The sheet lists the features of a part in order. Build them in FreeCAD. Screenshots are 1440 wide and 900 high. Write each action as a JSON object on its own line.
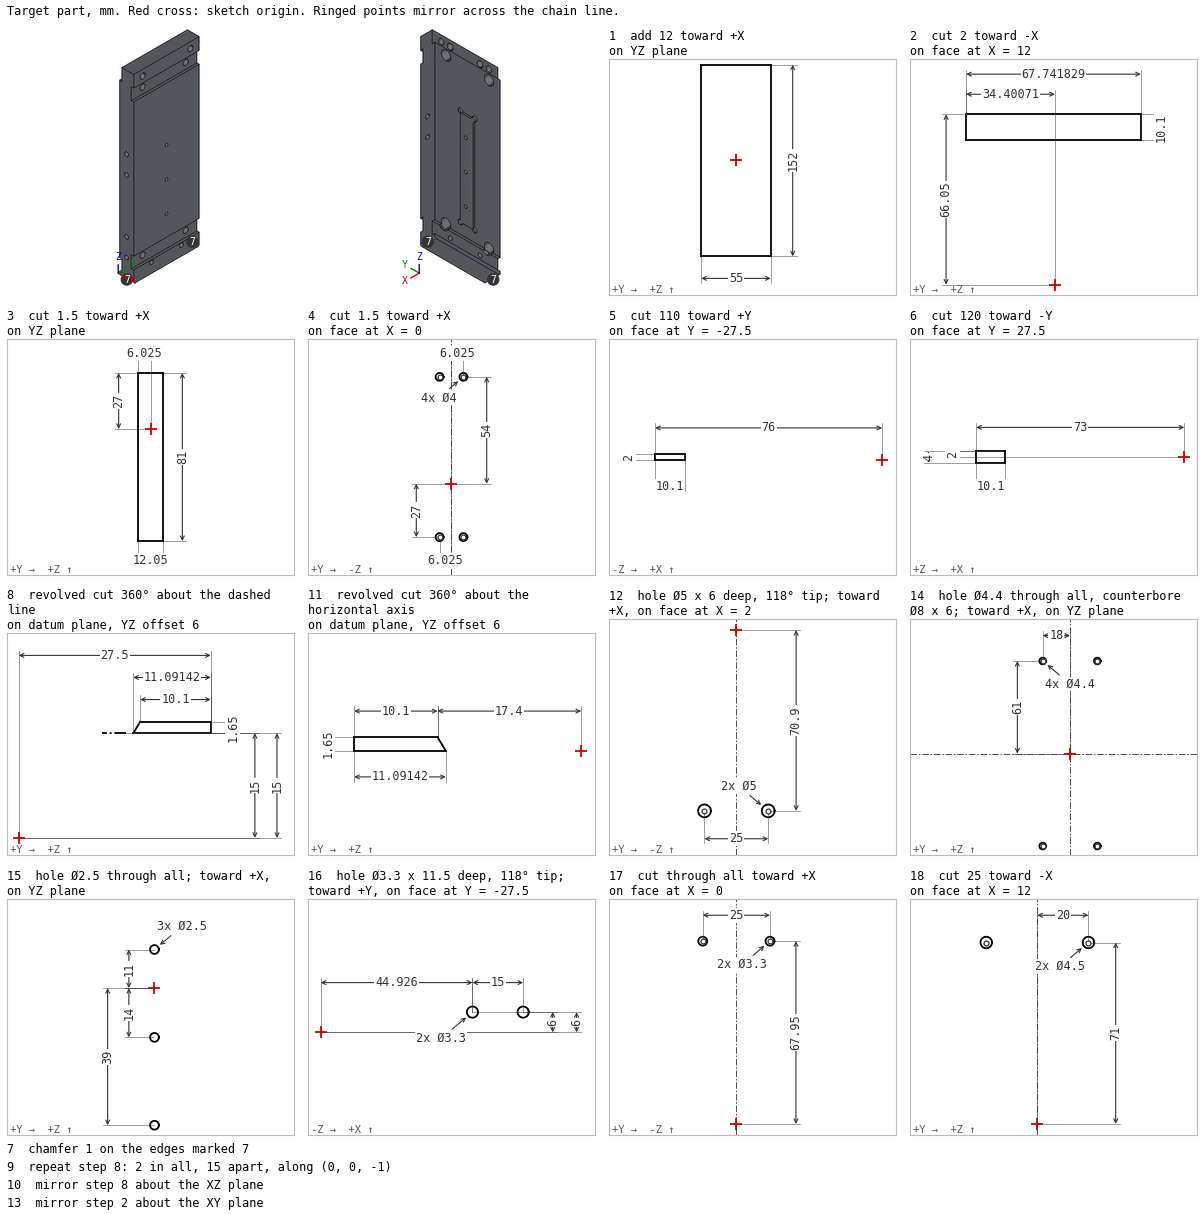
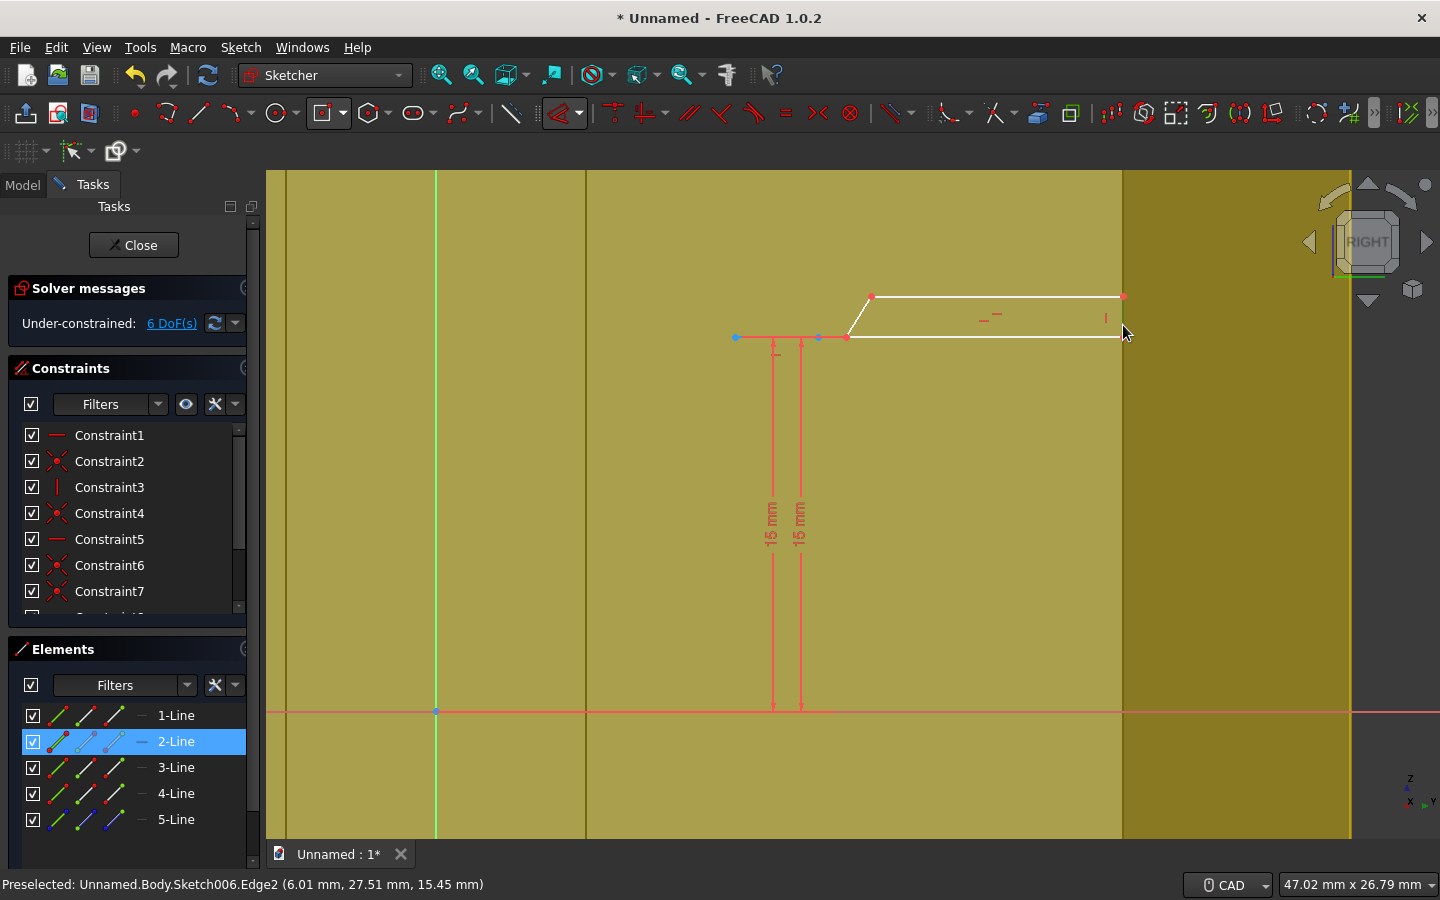
{"action": "left_click", "coordinate": [582, 114]}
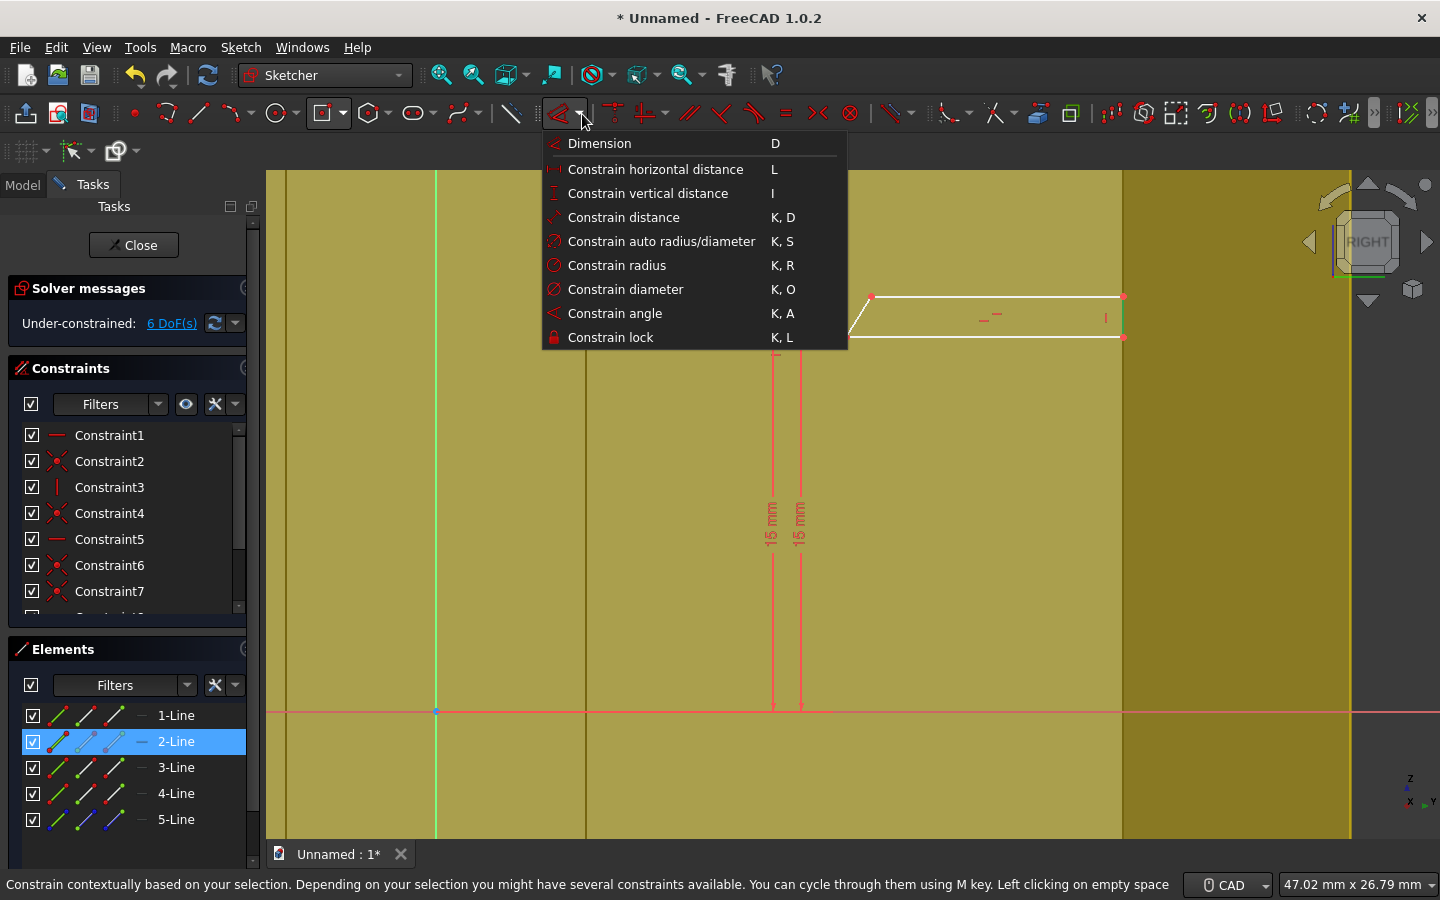
{"action": "left_click", "coordinate": [695, 193]}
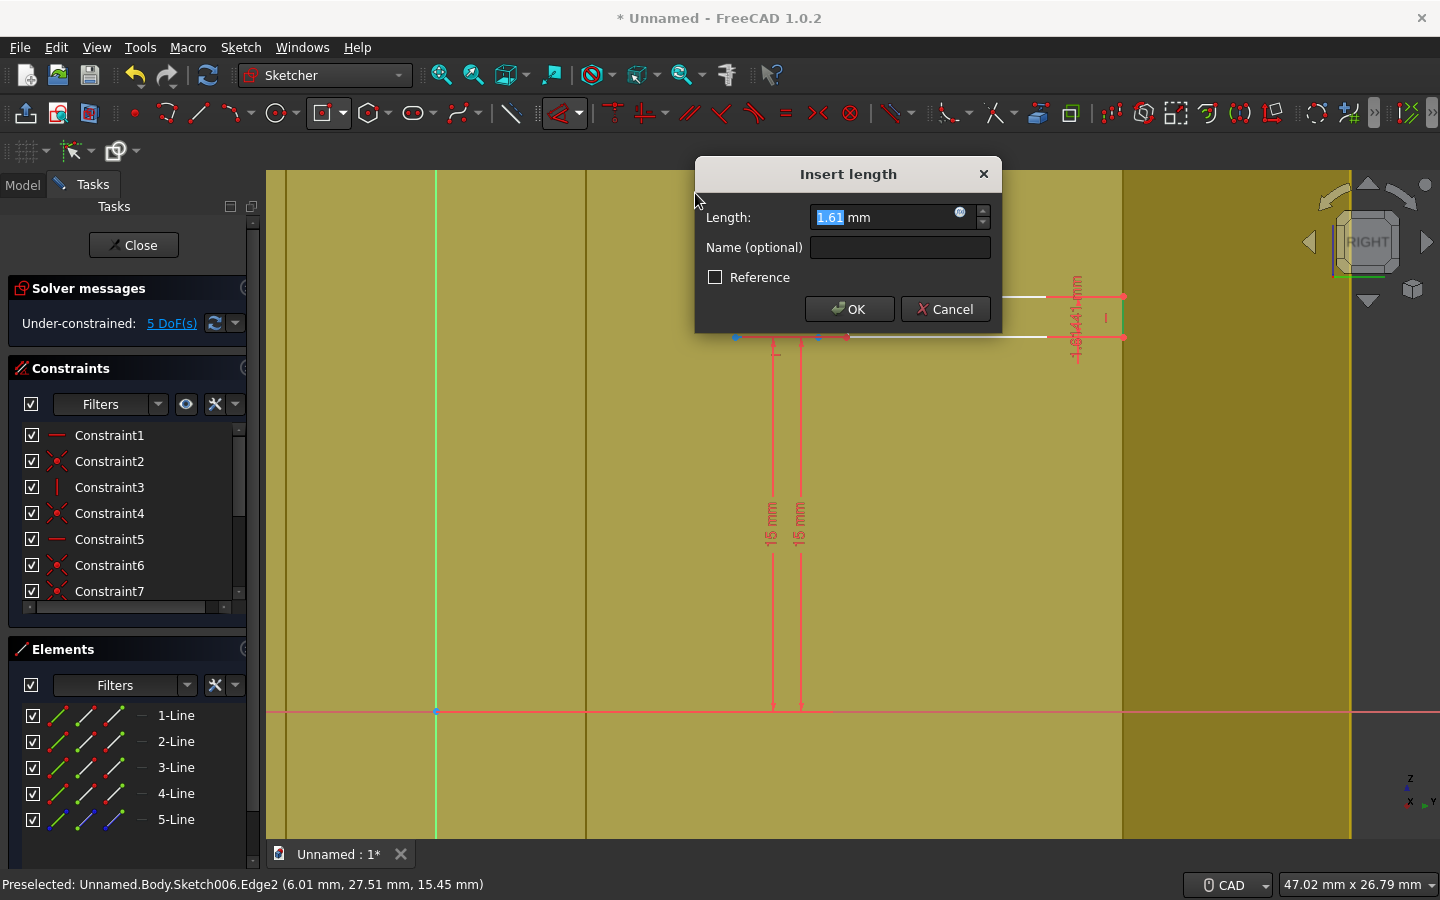
{"action": "type", "text": "1.65"}
{"action": "key", "text": "Return"}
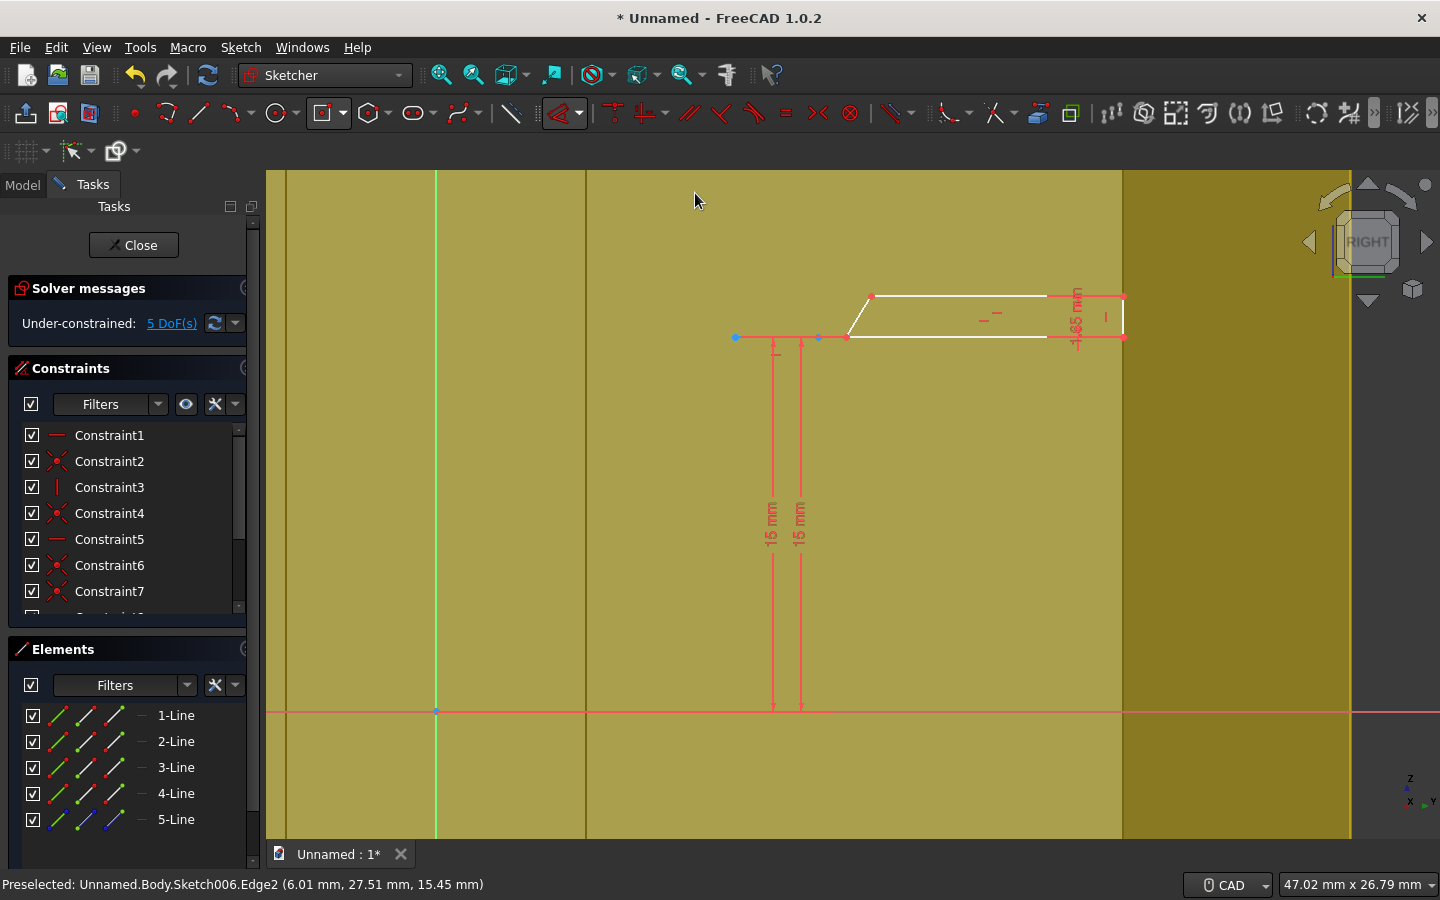
{"action": "left_click", "coordinate": [1047, 296]}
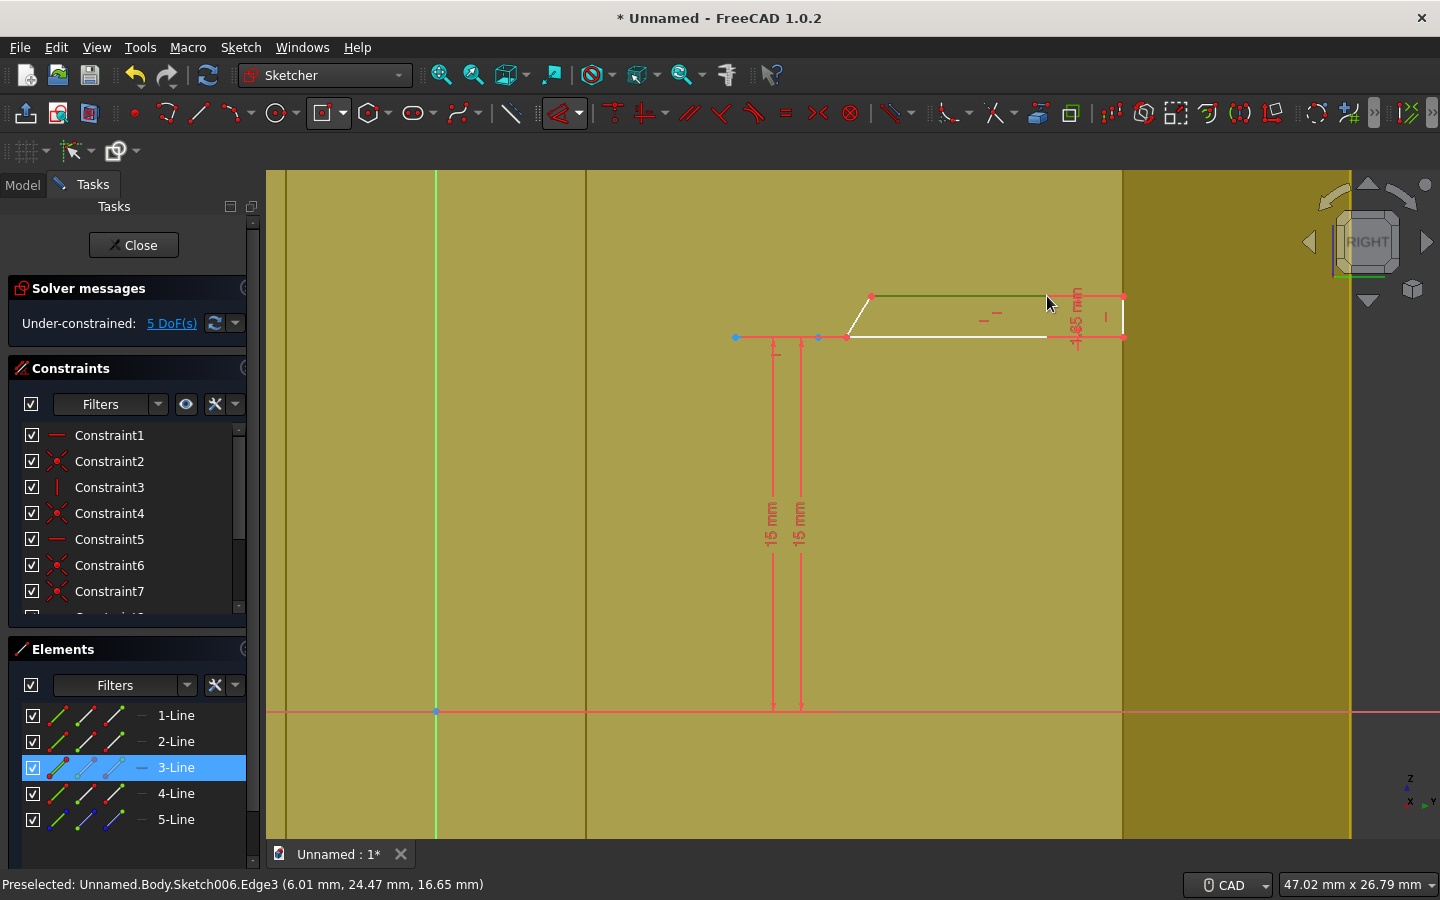
{"action": "key", "text": "l"}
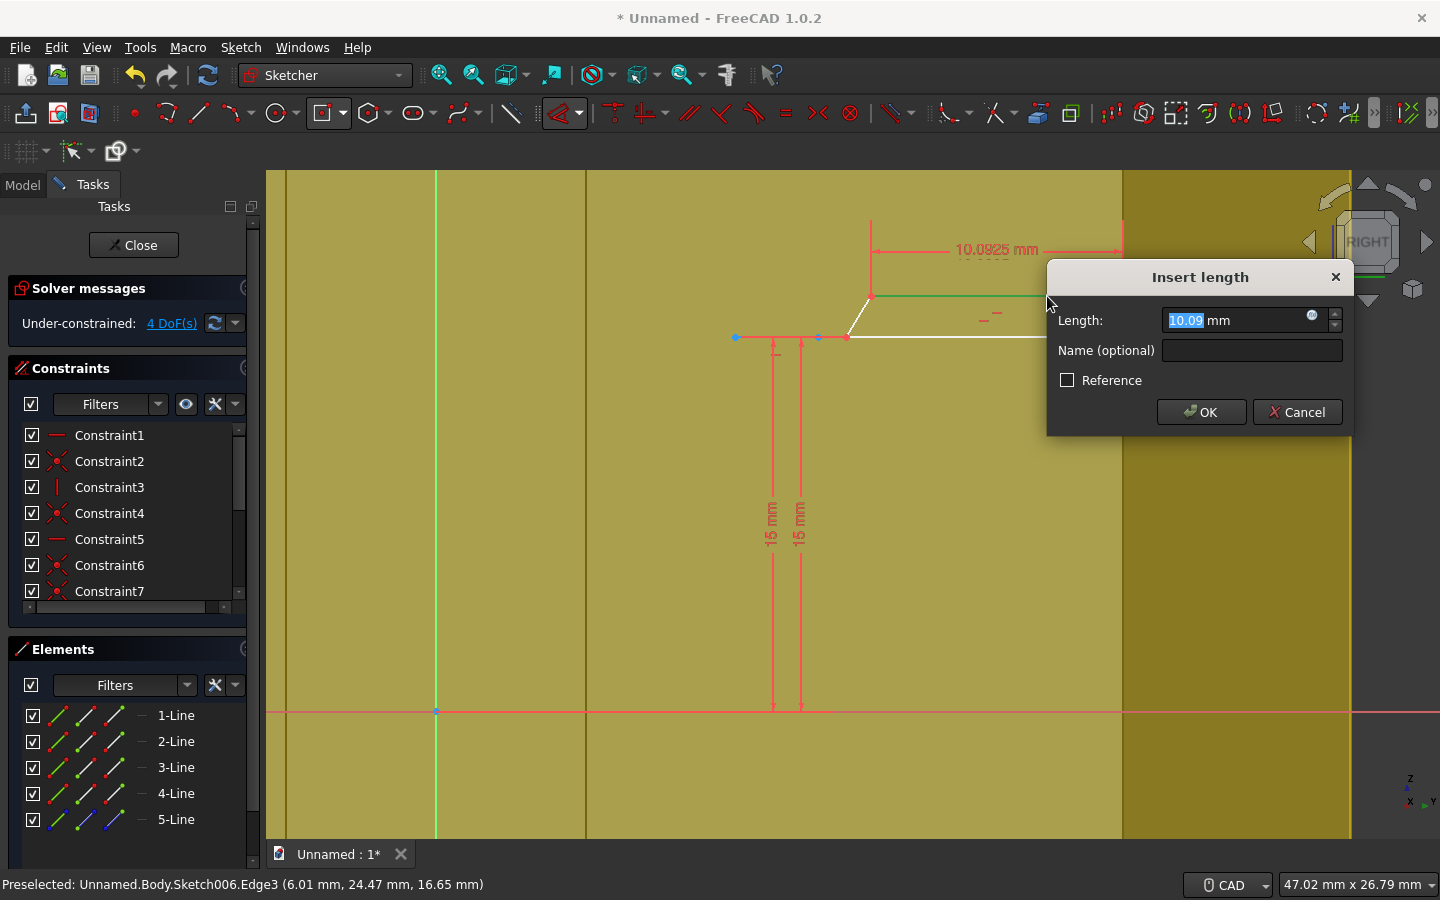
{"action": "type", "text": "10.1"}
{"action": "key", "text": "Return"}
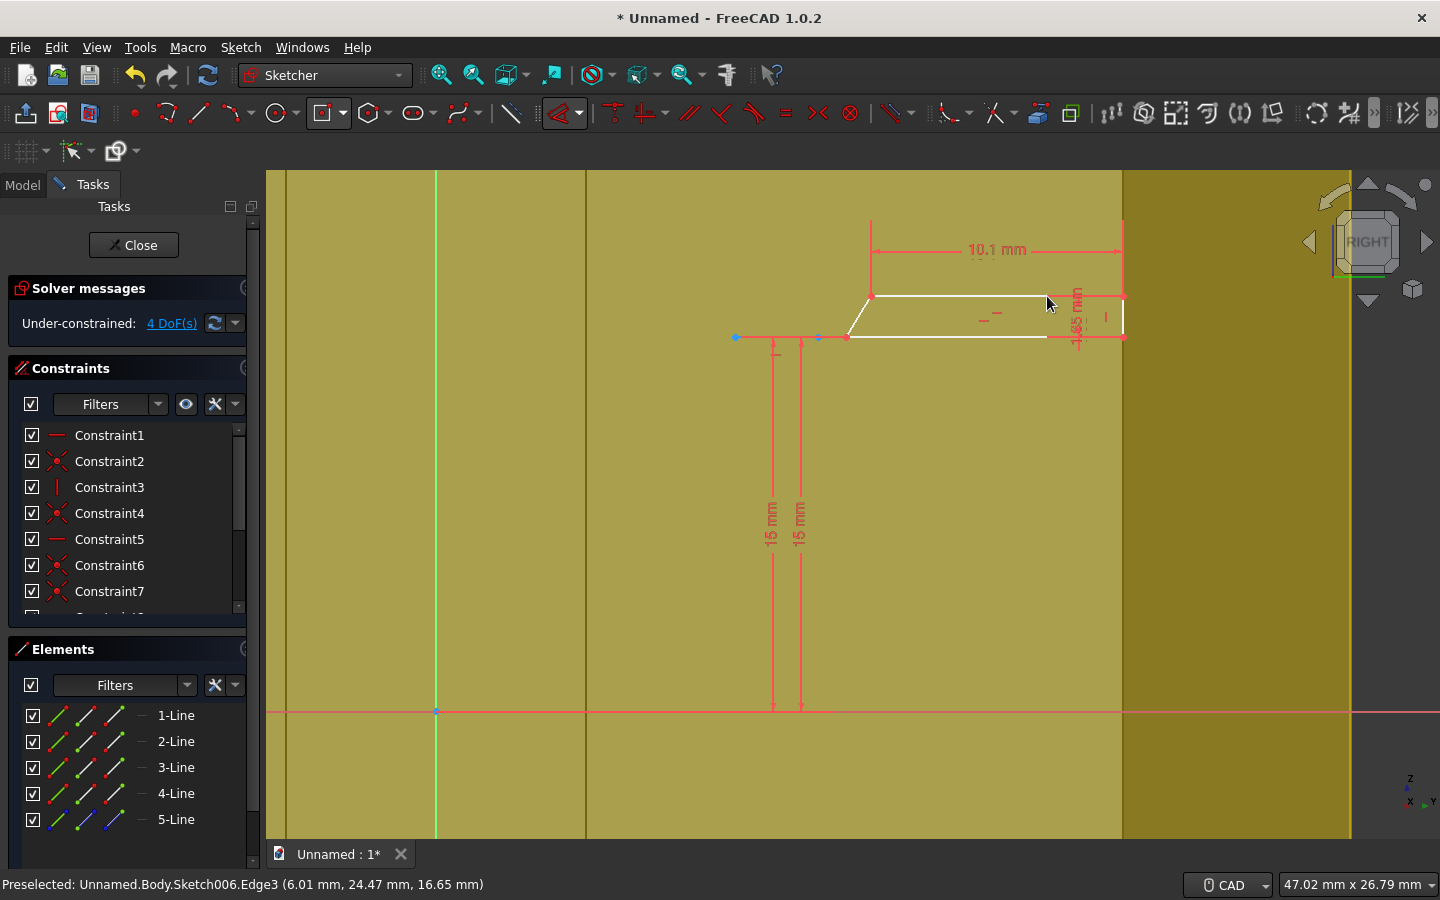
{"action": "left_click", "coordinate": [1123, 337]}